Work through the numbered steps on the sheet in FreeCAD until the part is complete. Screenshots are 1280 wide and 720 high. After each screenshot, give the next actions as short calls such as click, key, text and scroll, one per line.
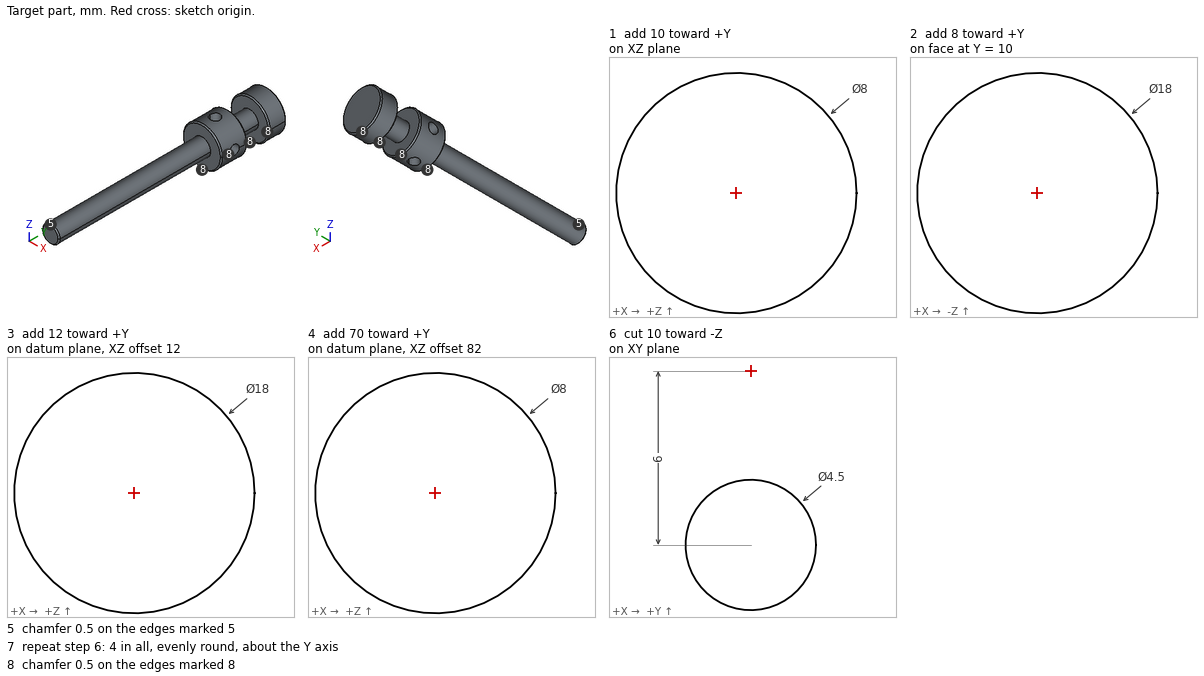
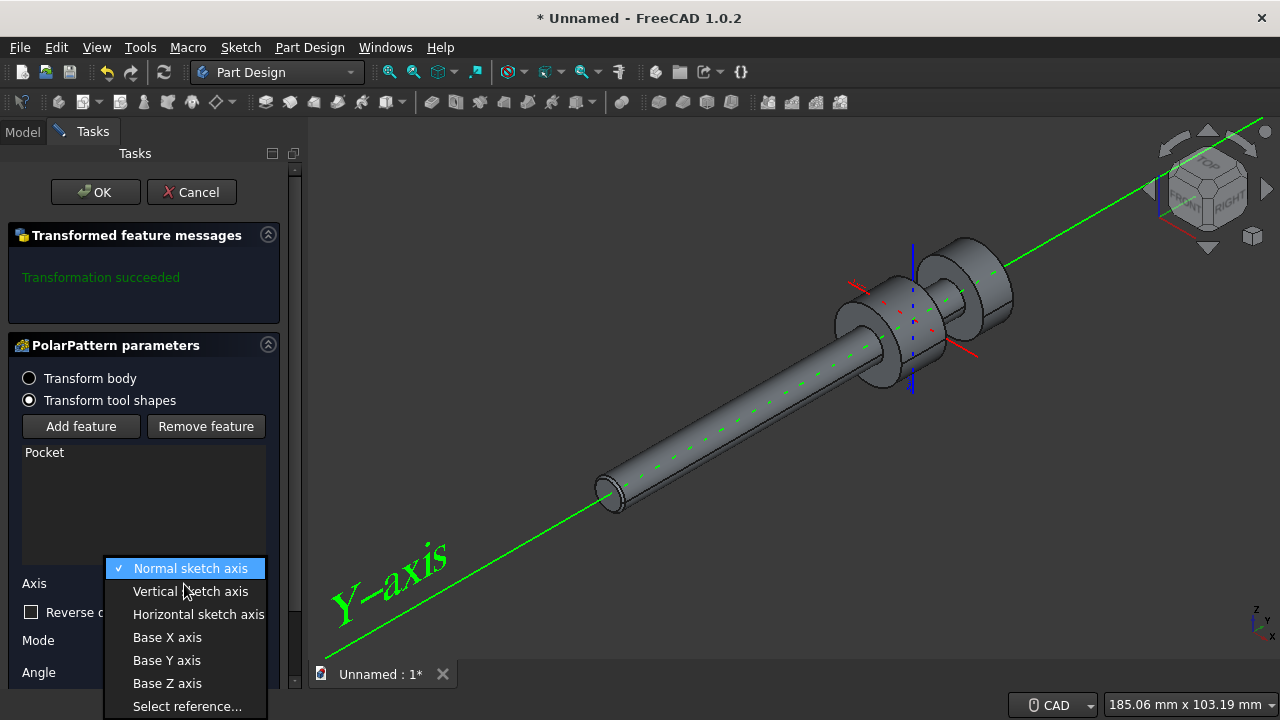
click(184, 660)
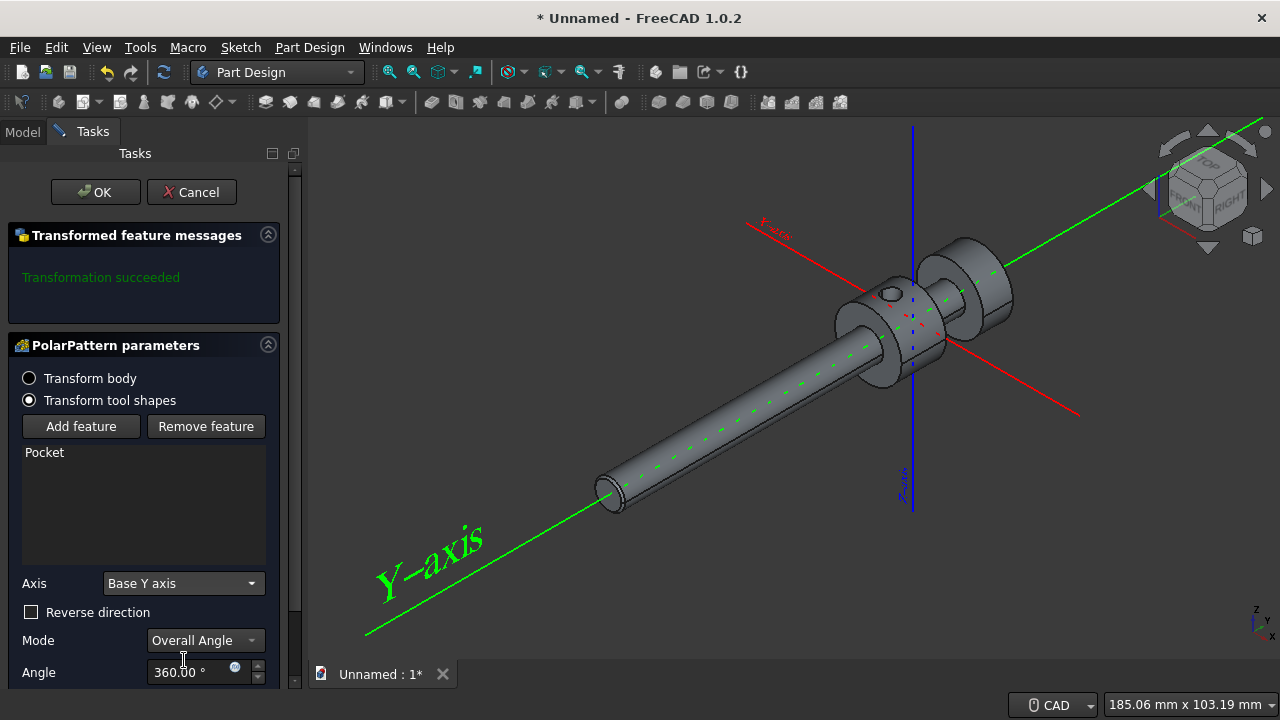
scroll(295, 426, down, 2)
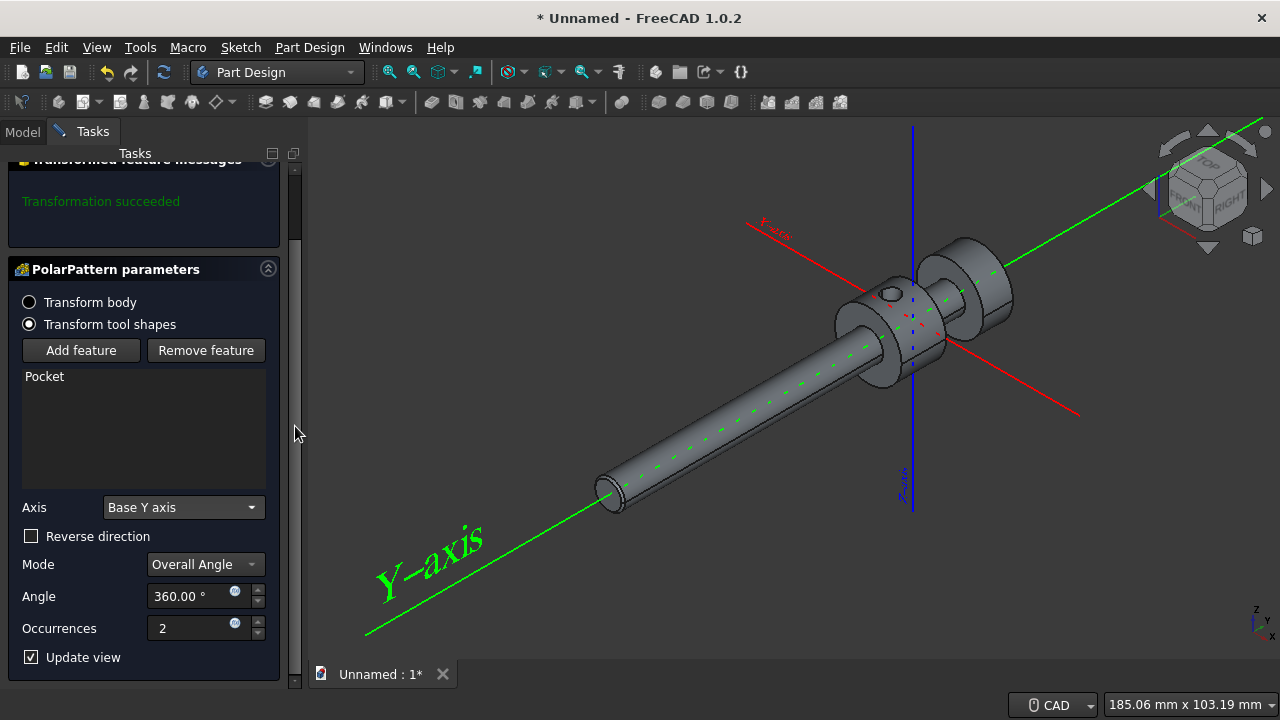
triple_click(198, 628)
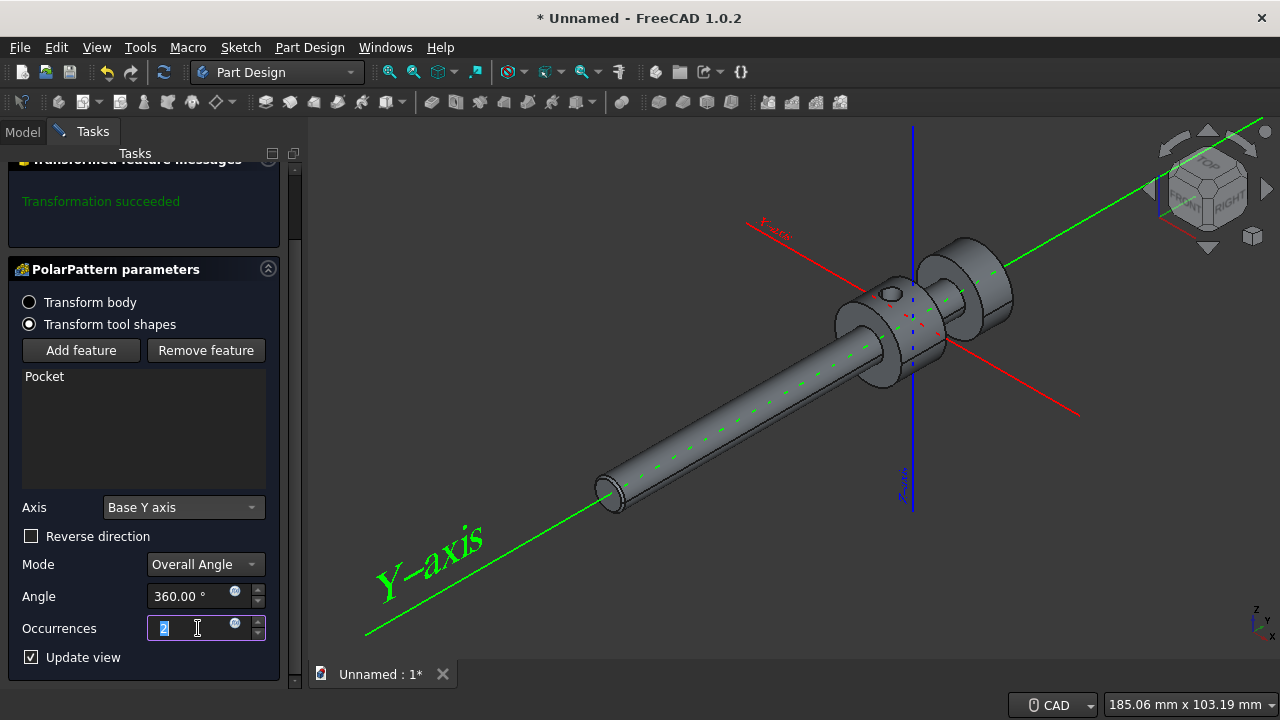
text(4)
key(Tab)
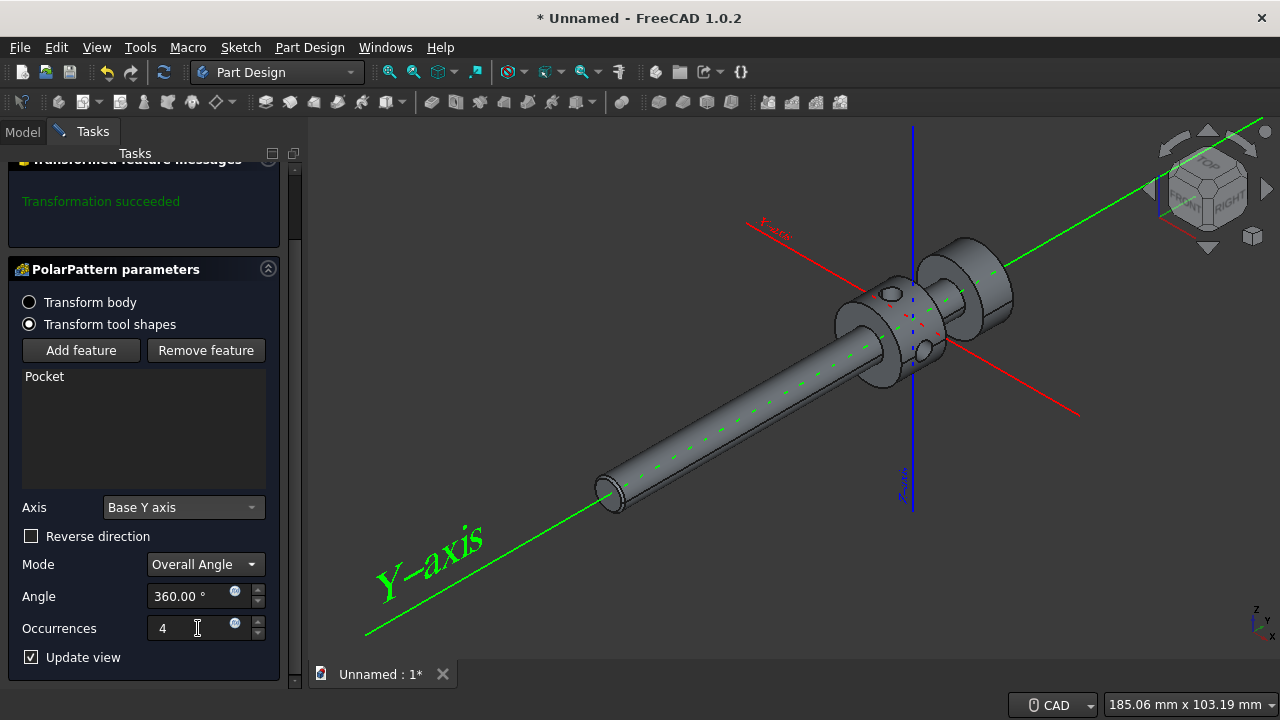
scroll(295, 426, up, 3)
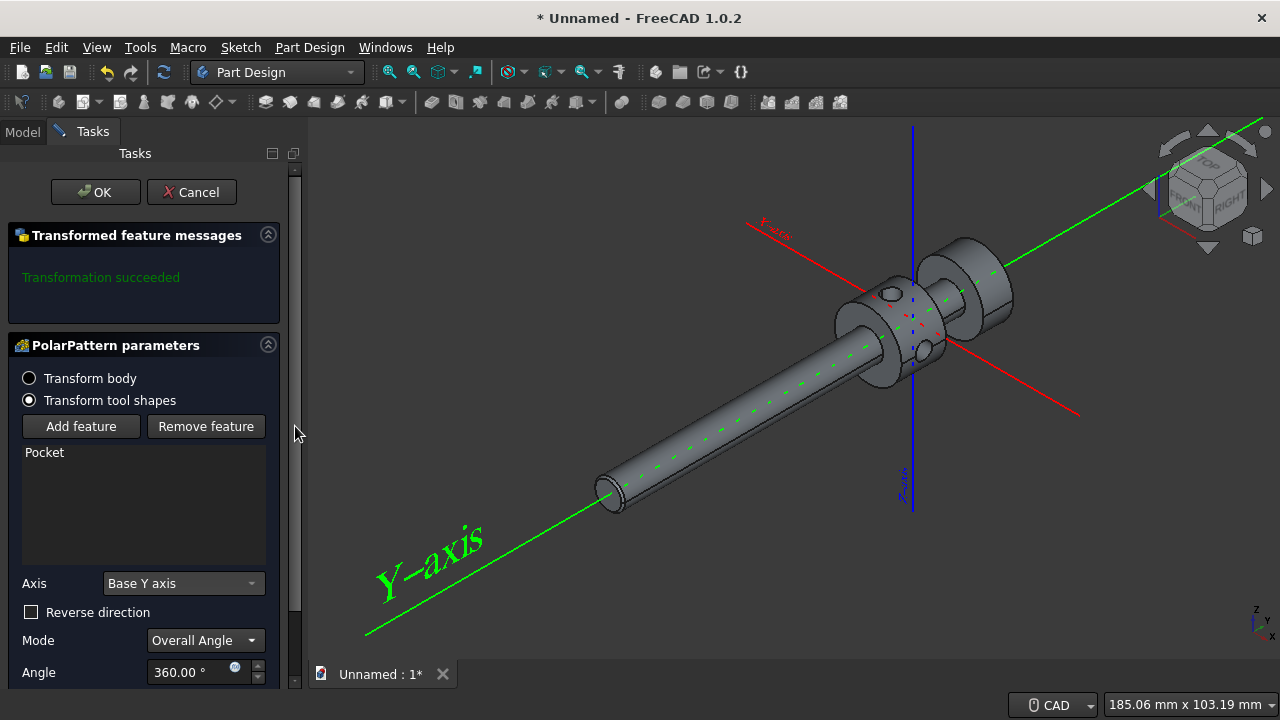
click(96, 192)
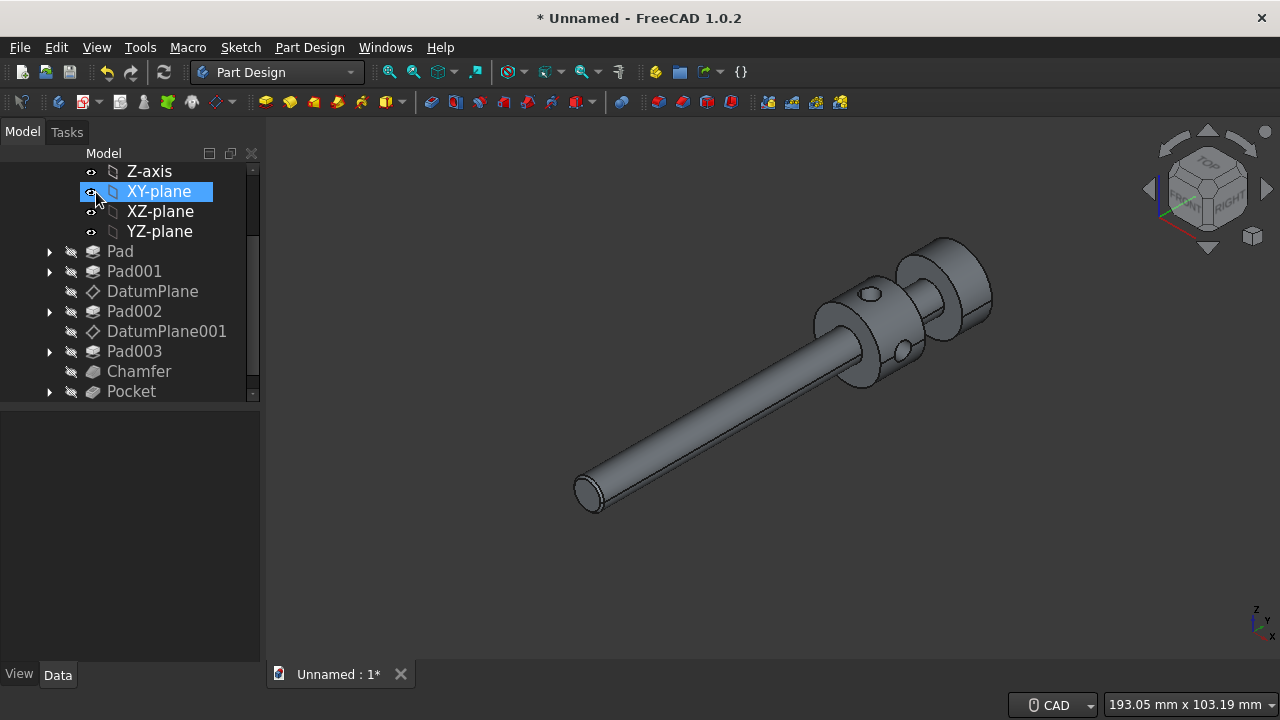
click(919, 254)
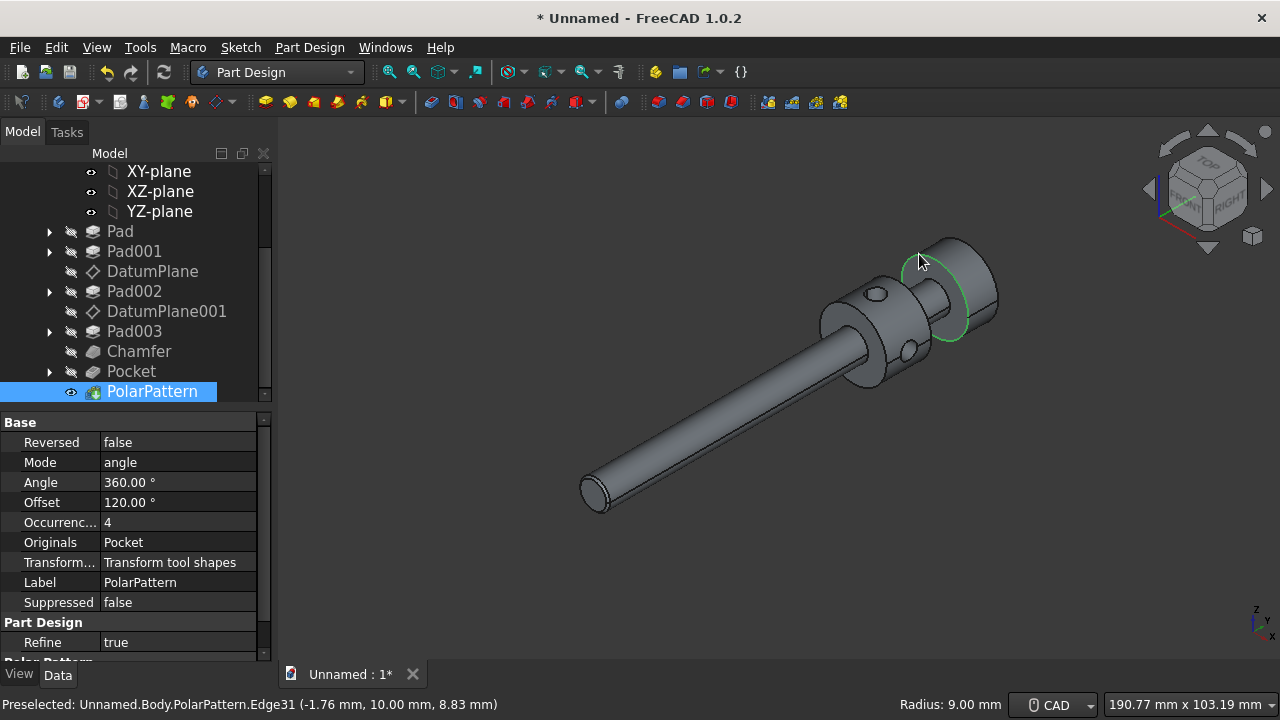
click(975, 249, ctrl)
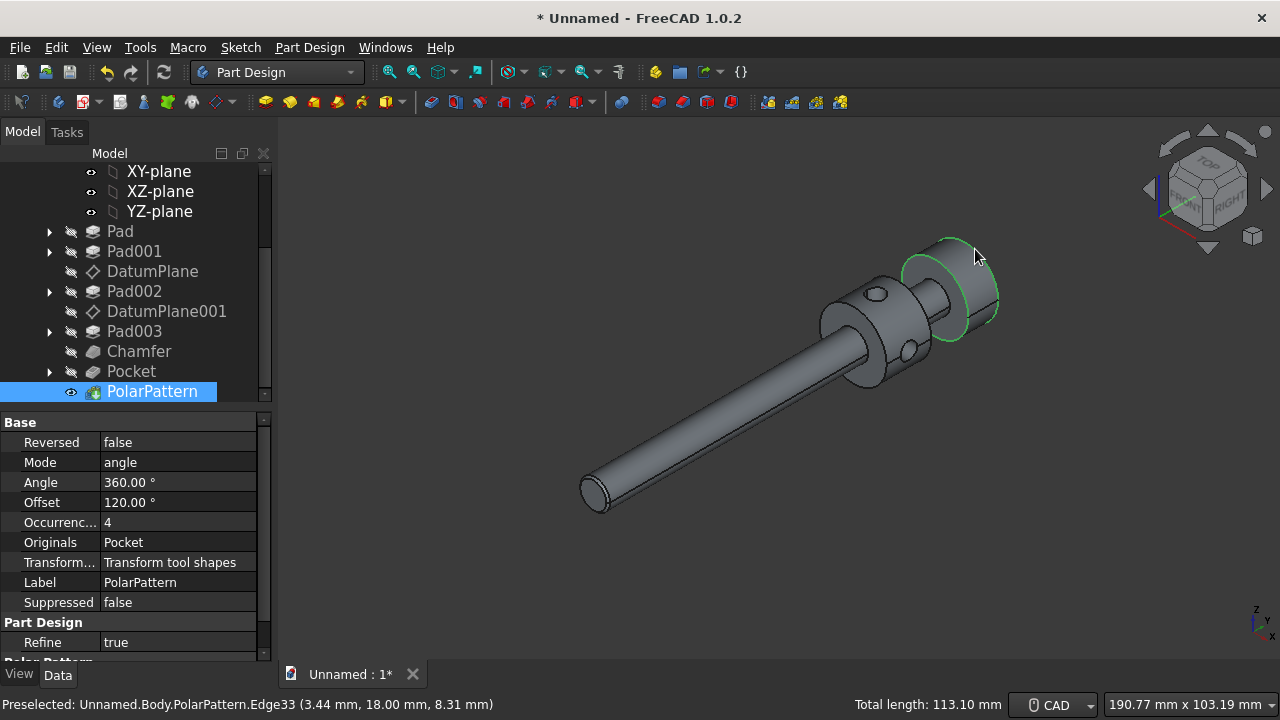
click(843, 301, ctrl)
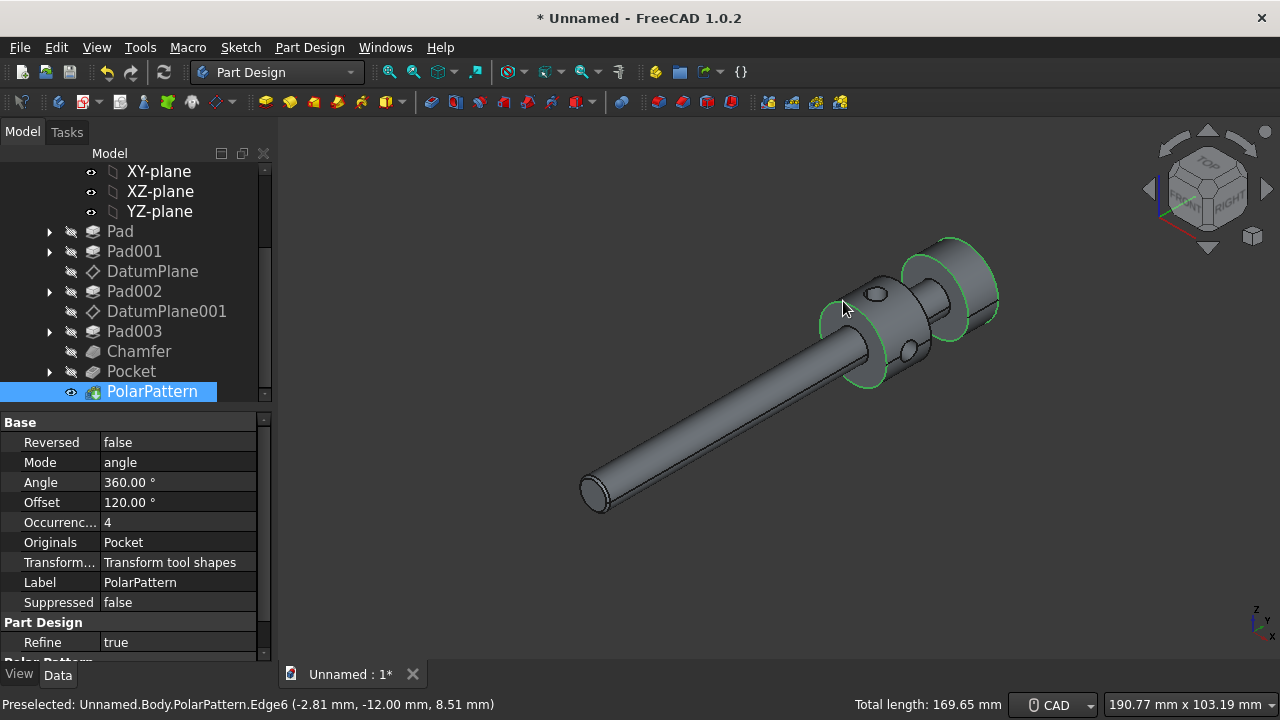
key(2)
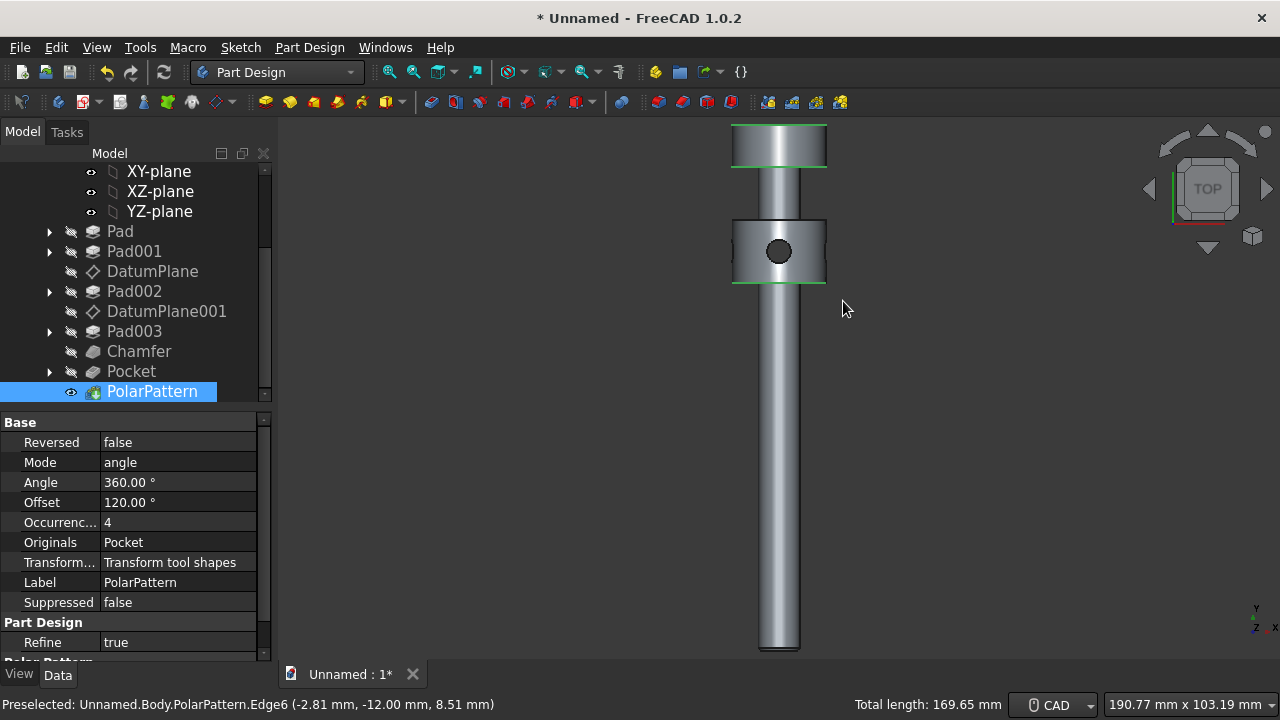
click(741, 219, ctrl)